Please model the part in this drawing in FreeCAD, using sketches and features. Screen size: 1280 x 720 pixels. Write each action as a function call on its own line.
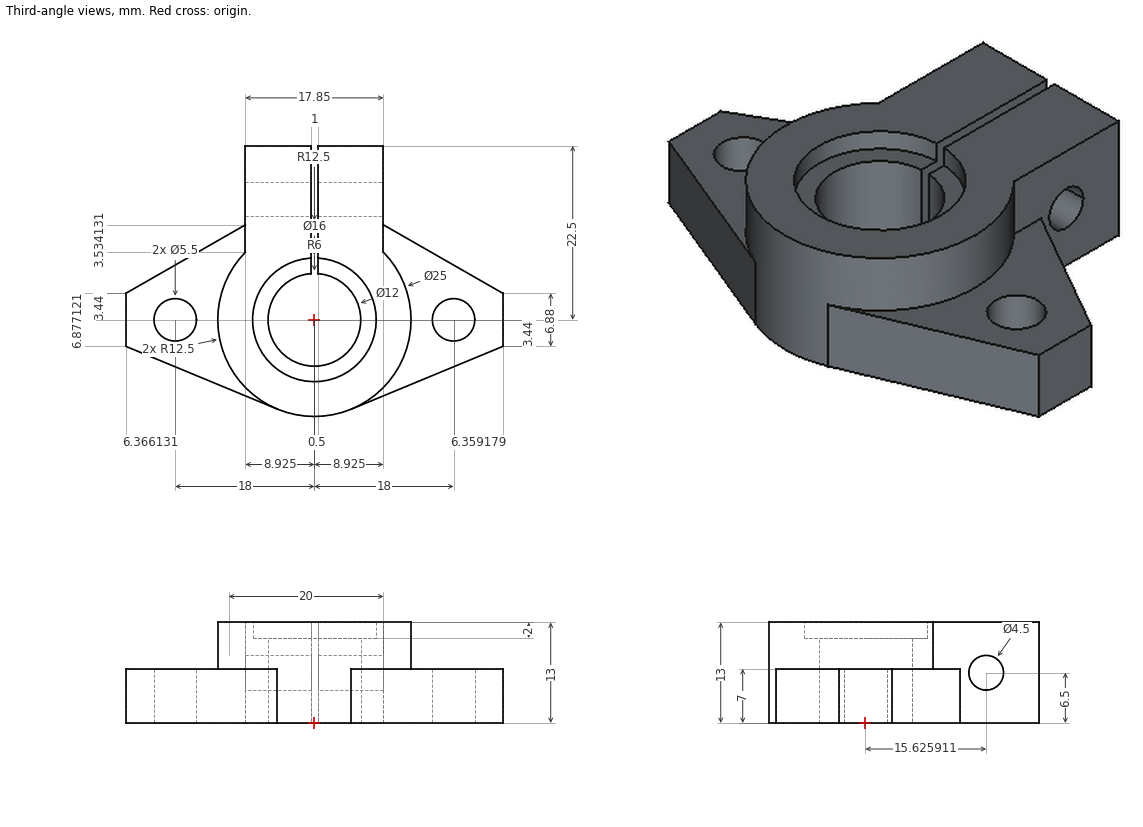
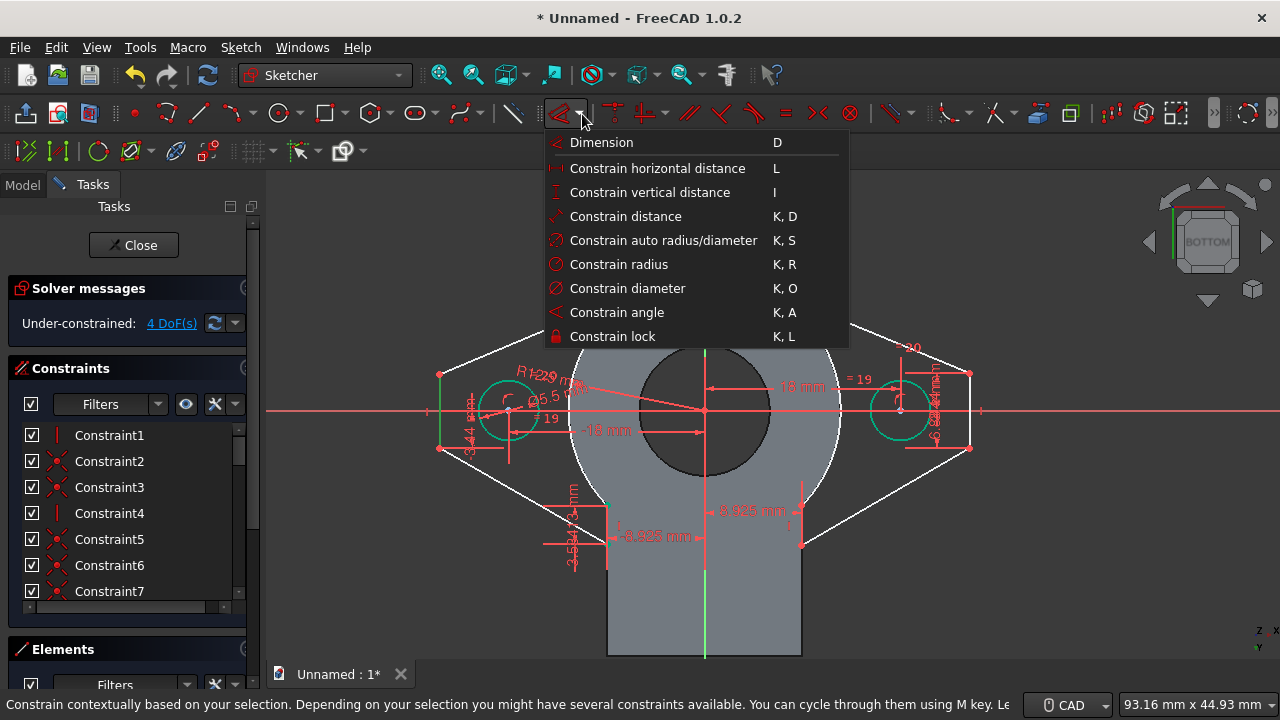
click(697, 192)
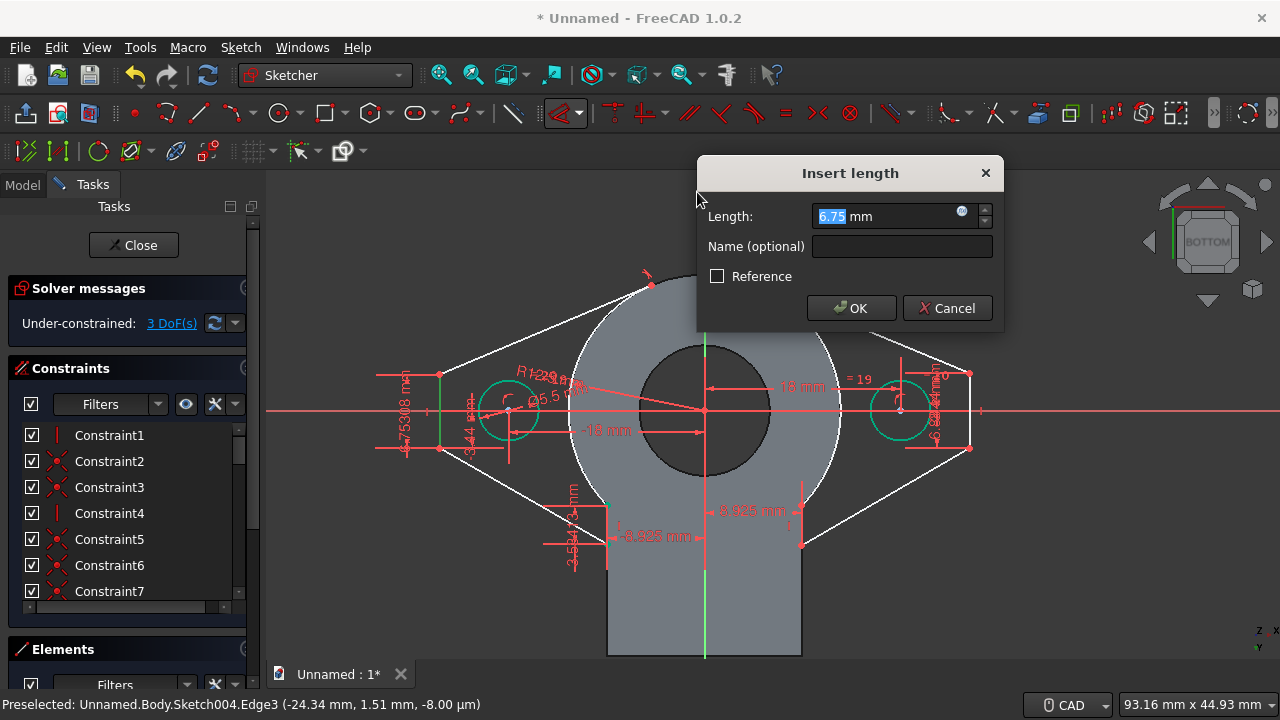
text(6.877121)
key(Return)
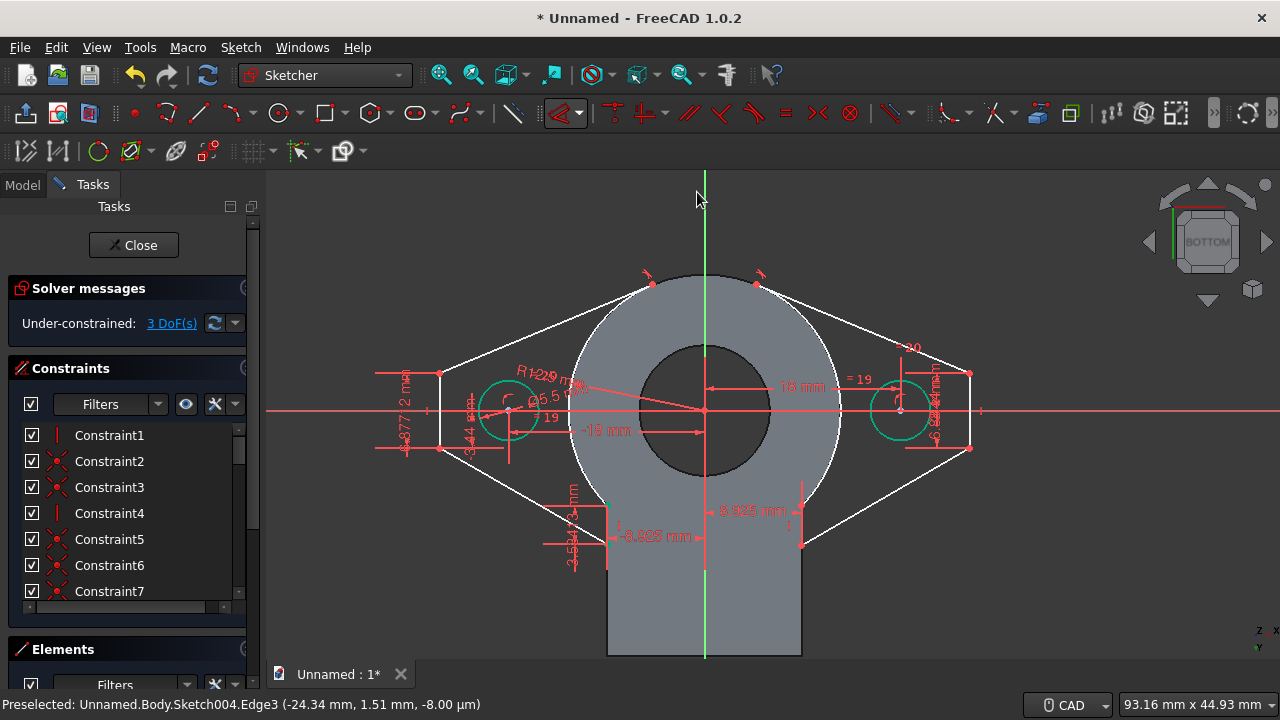
scroll(802, 534, up, 2)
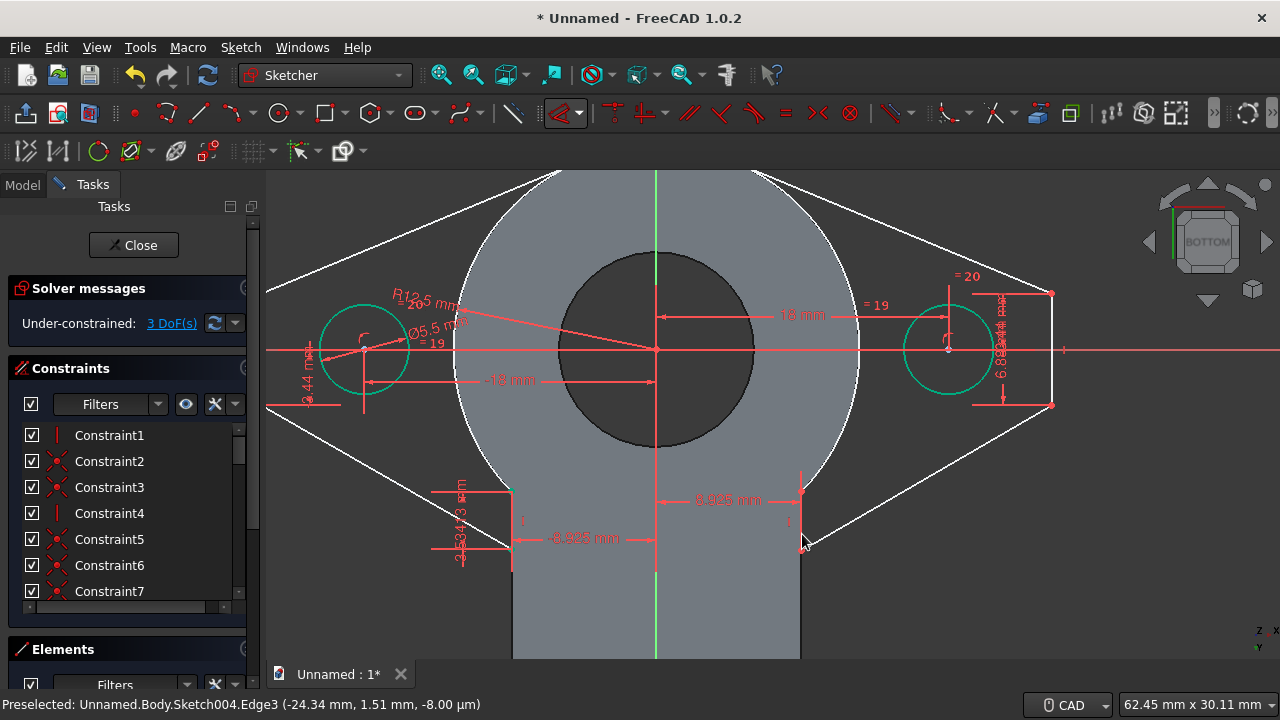
click(801, 533)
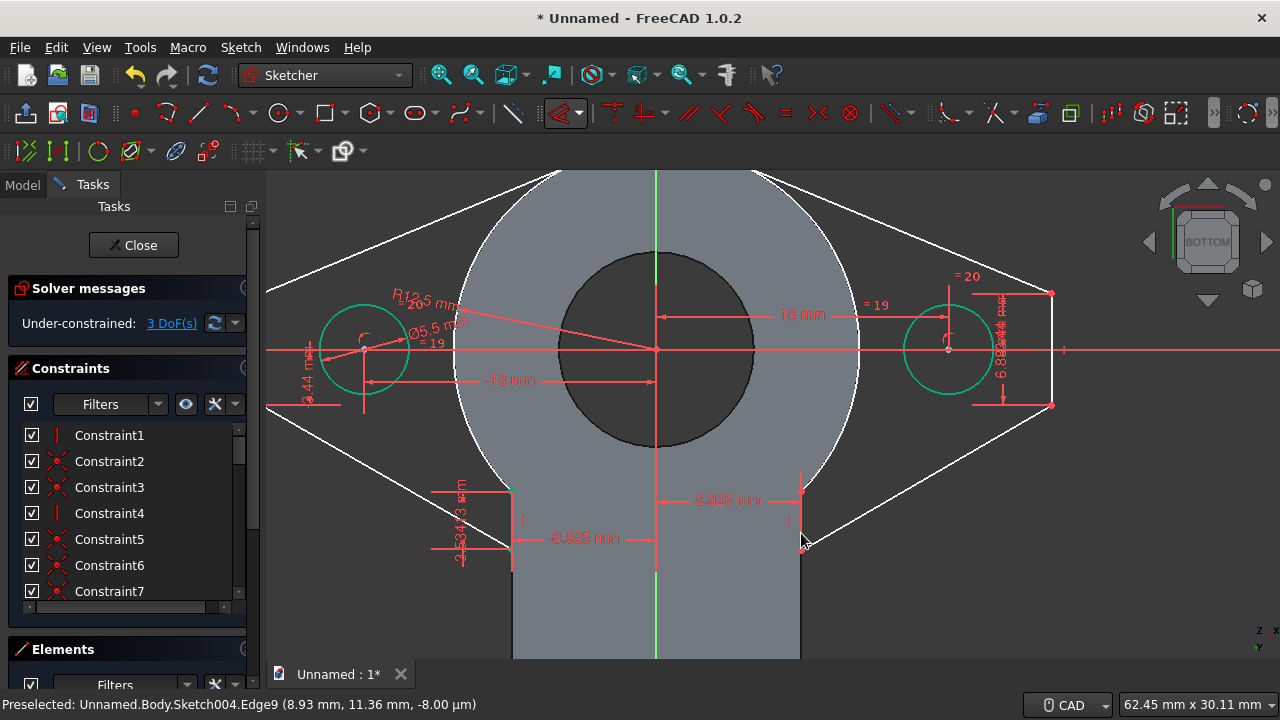
click(582, 114)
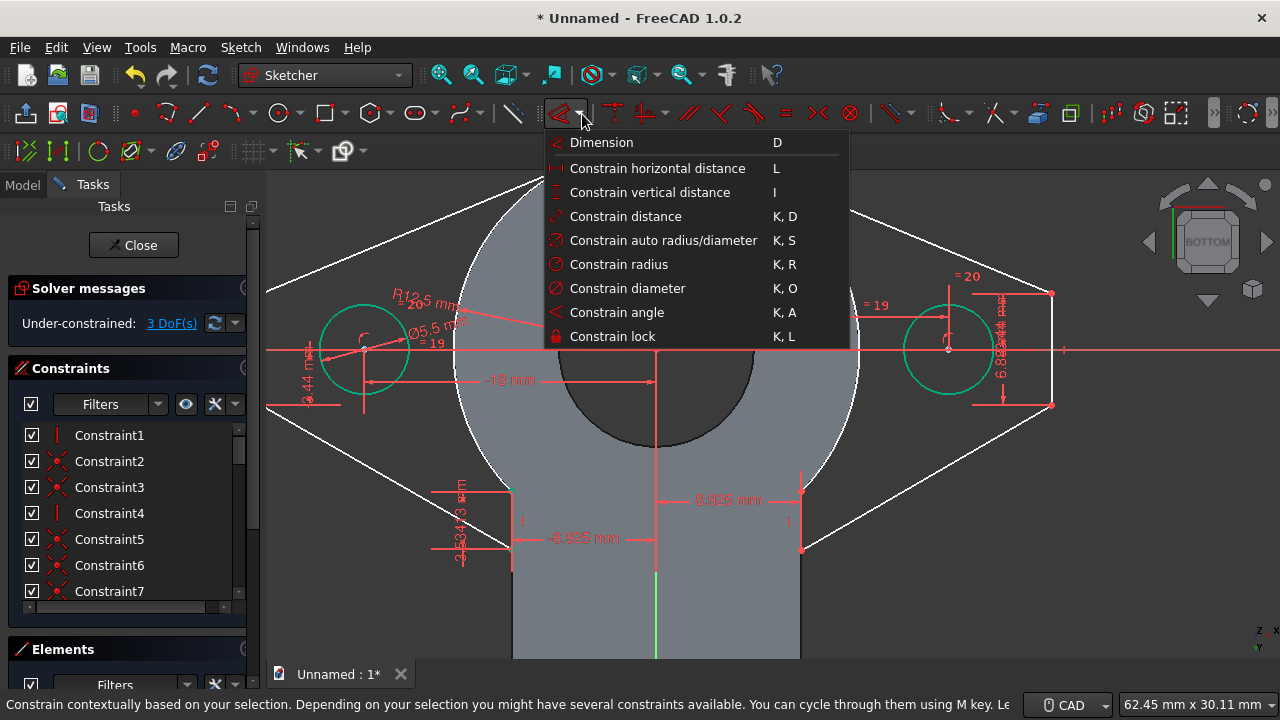
click(697, 192)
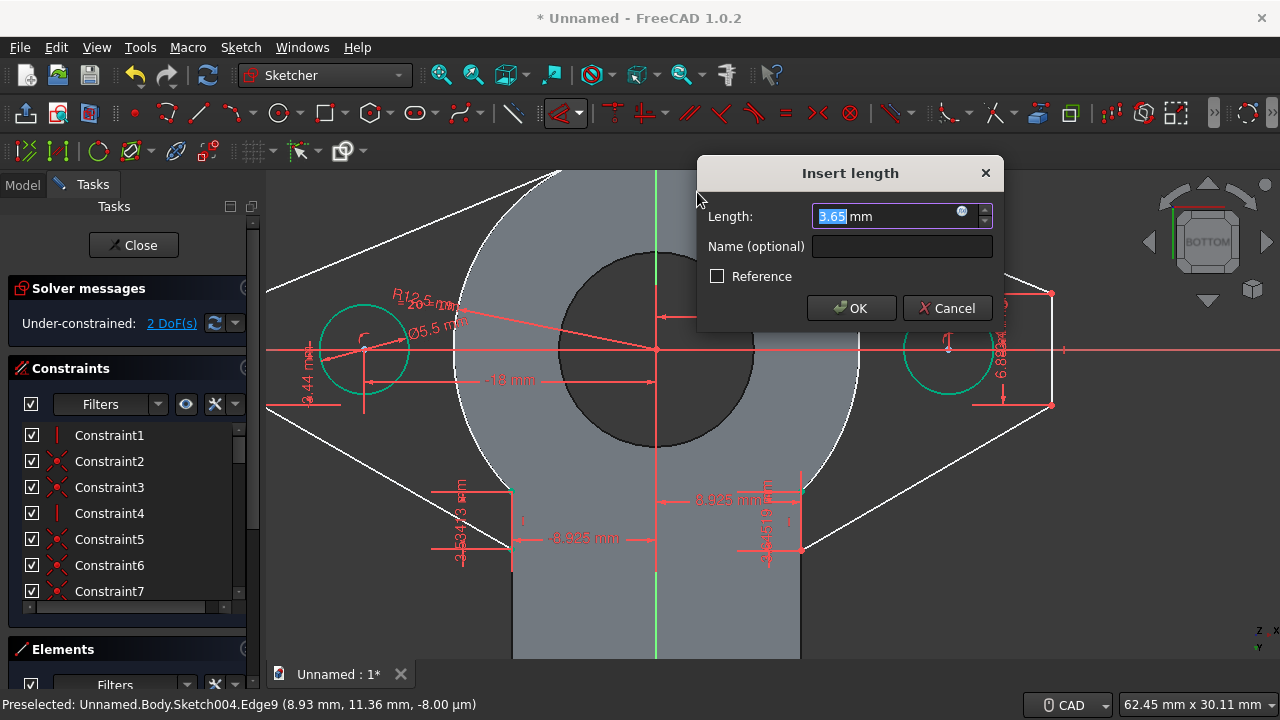
text(3.534131)
key(Return)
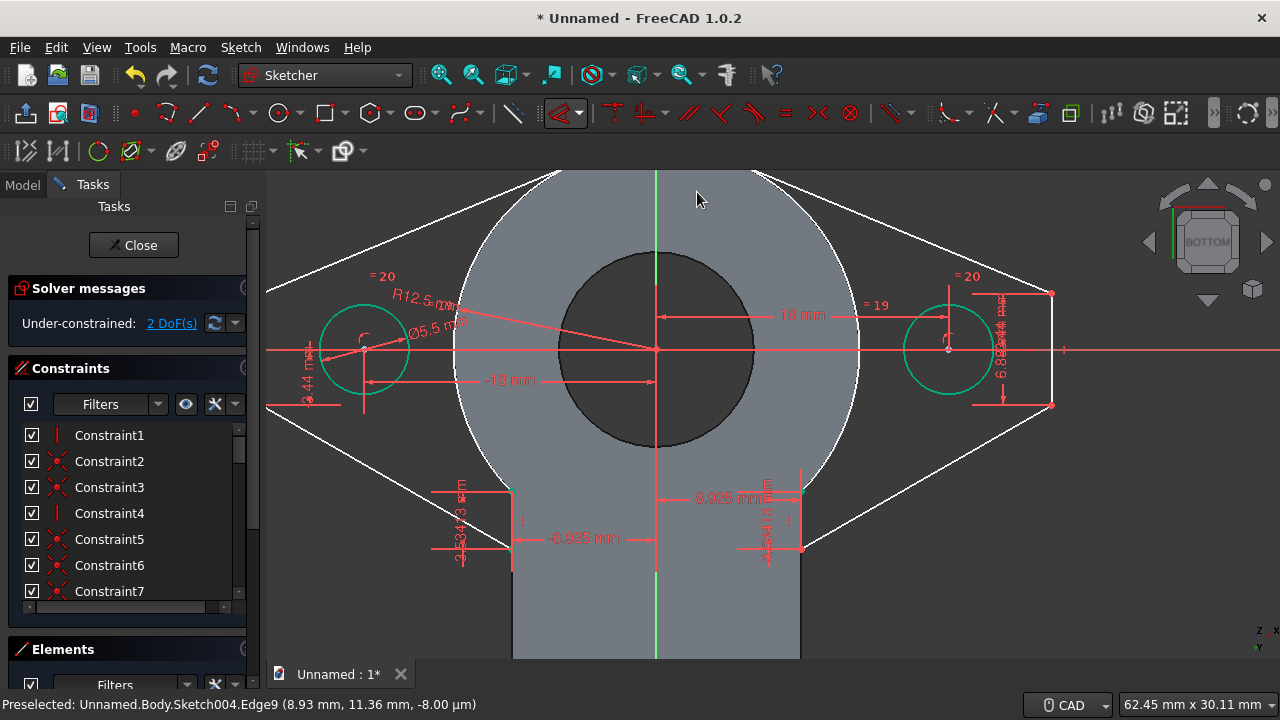
scroll(802, 534, down, 2)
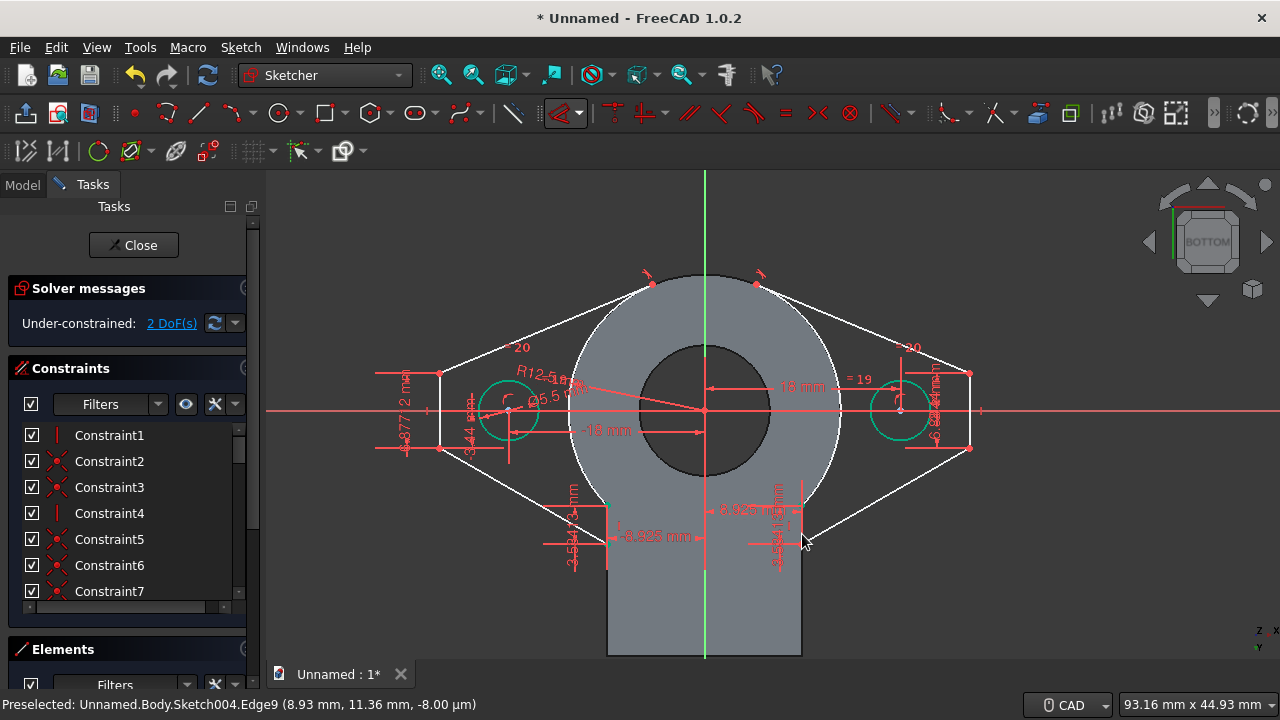
click(440, 373)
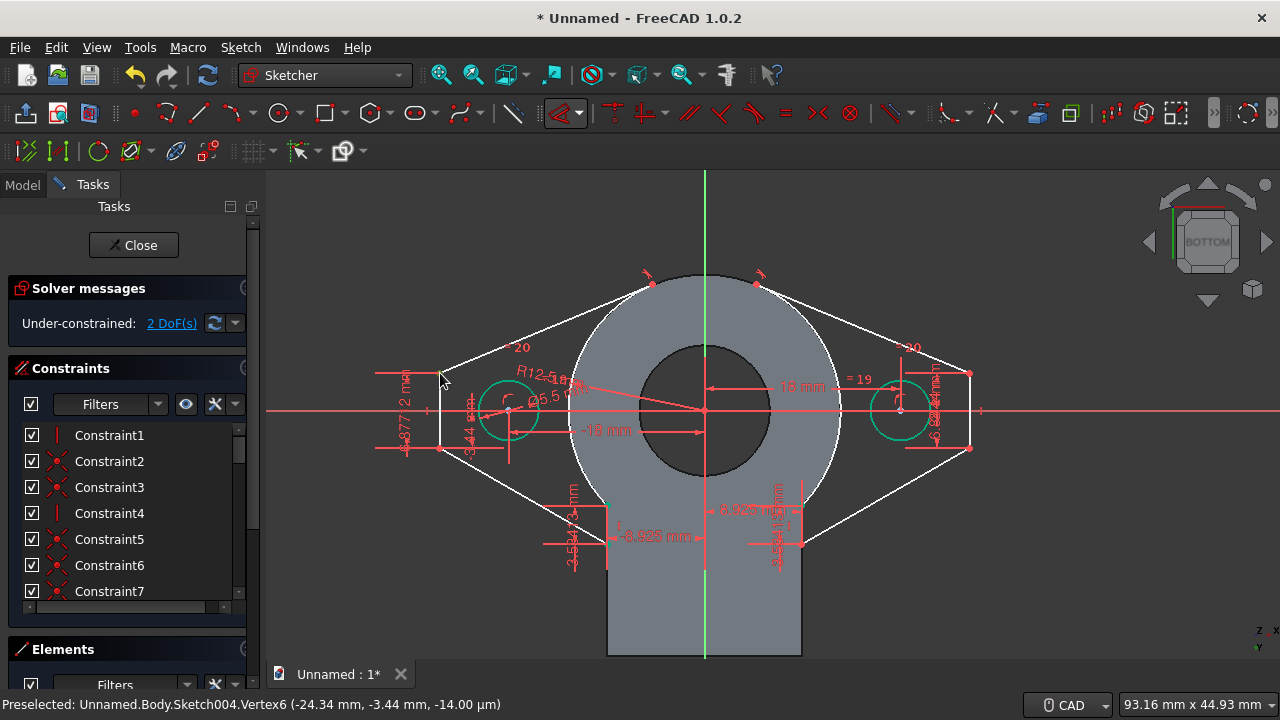
click(509, 411)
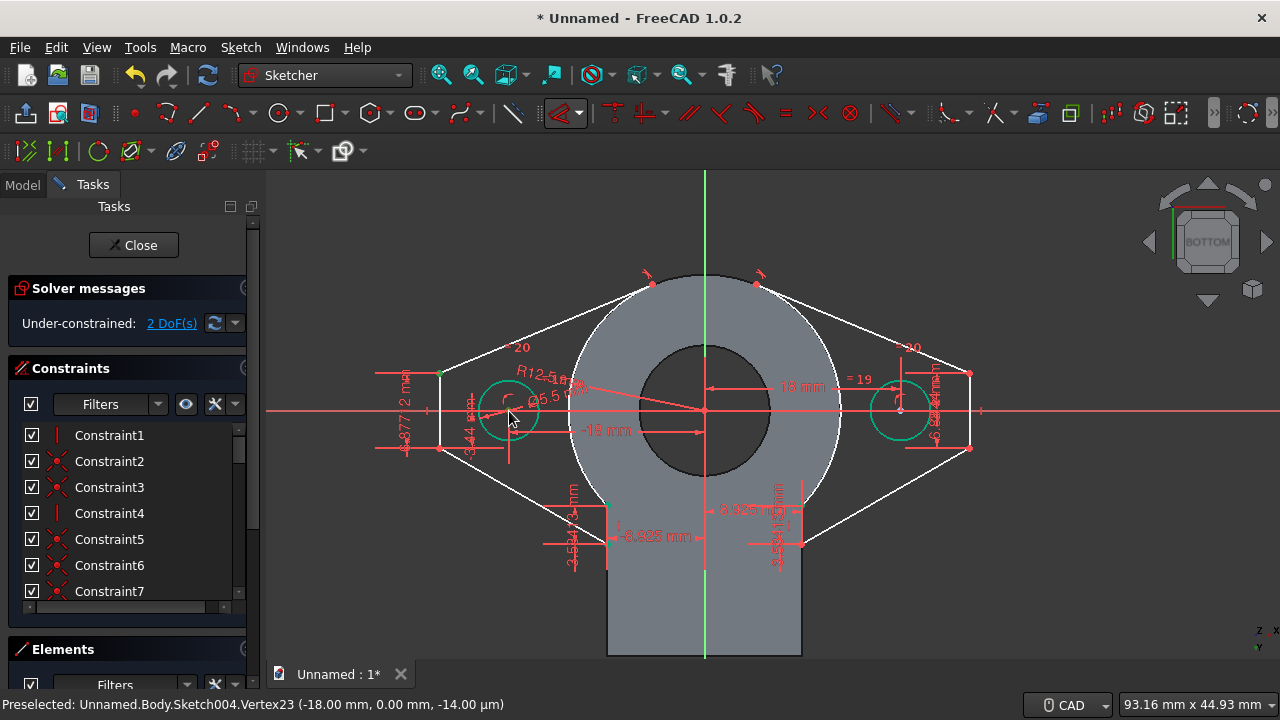
key(l)